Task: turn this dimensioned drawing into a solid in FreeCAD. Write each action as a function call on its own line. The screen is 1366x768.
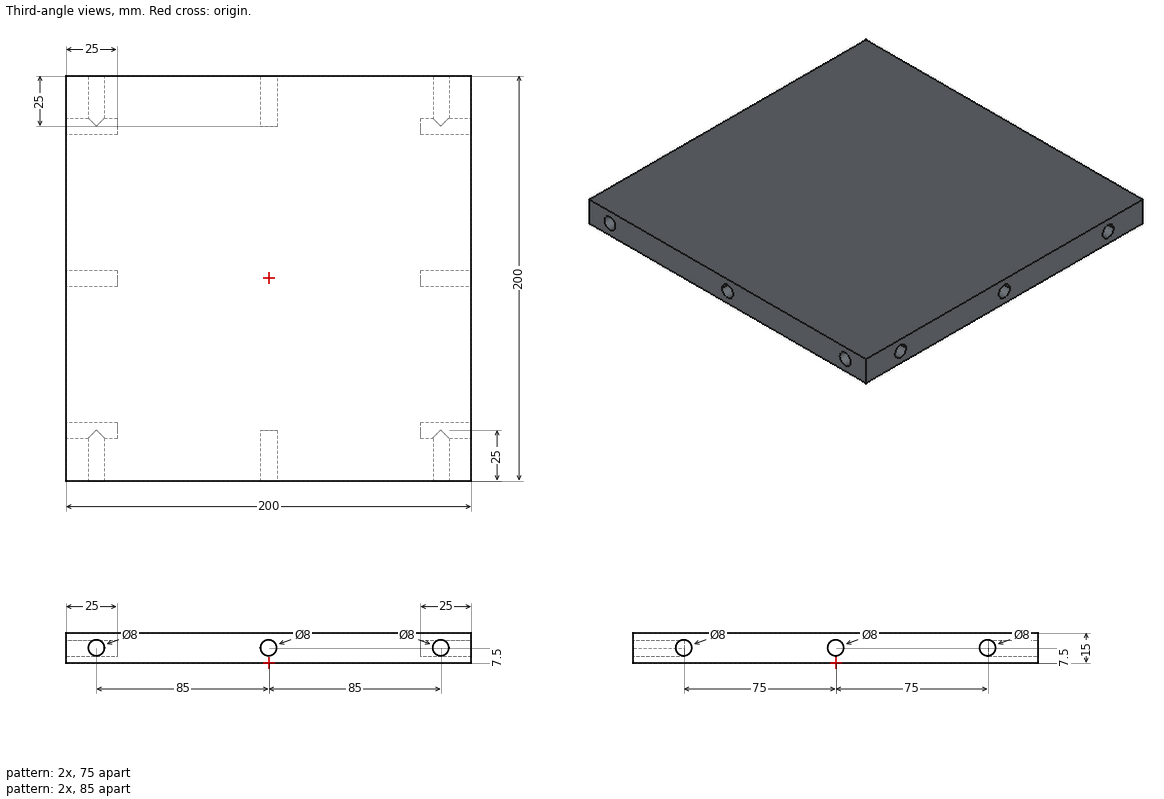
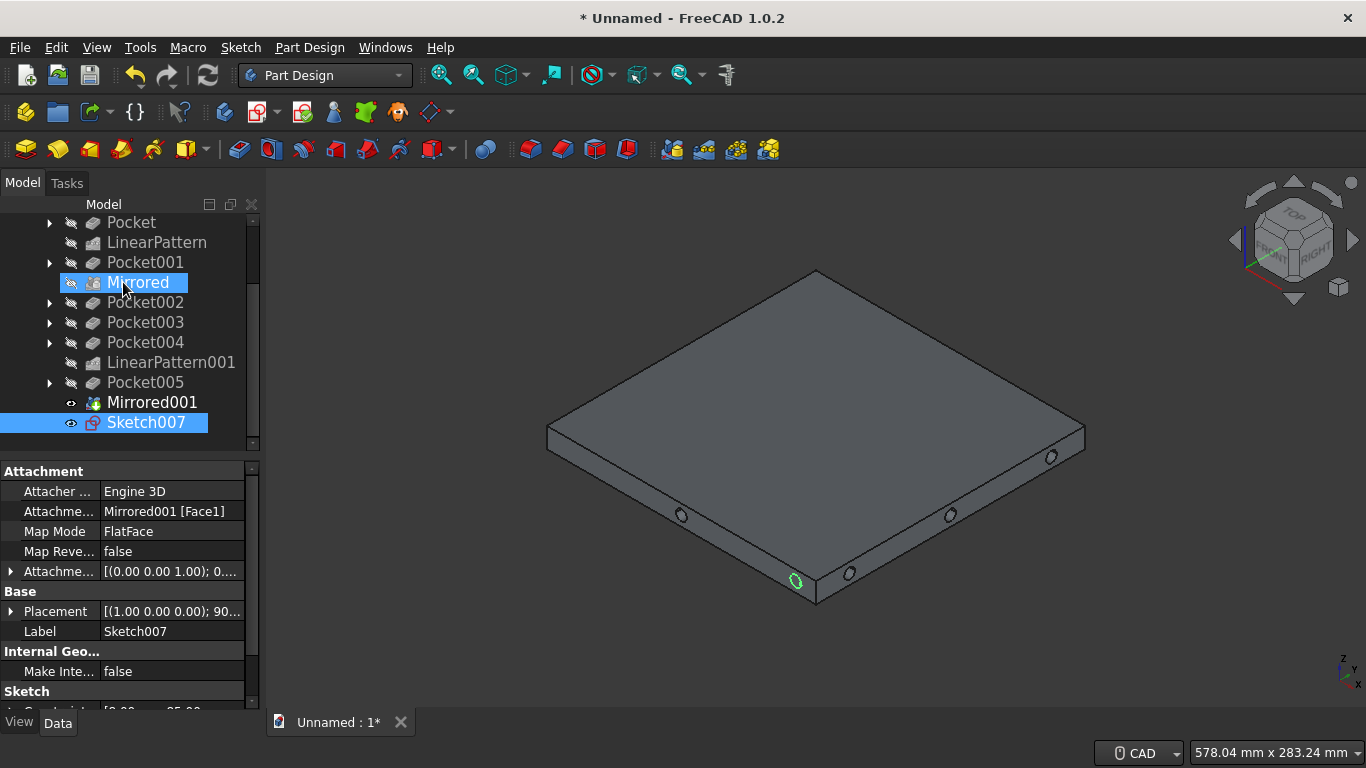
click(240, 150)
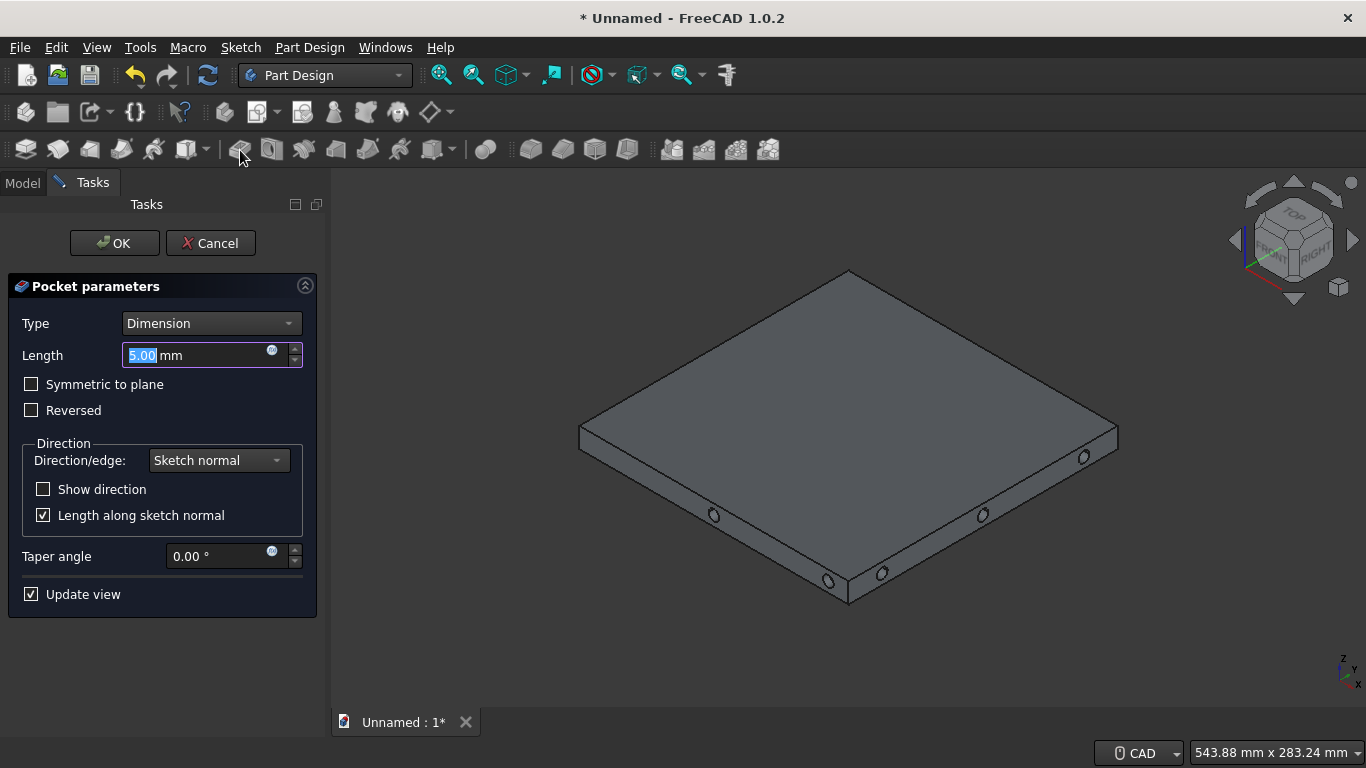
text(25)
key(Tab)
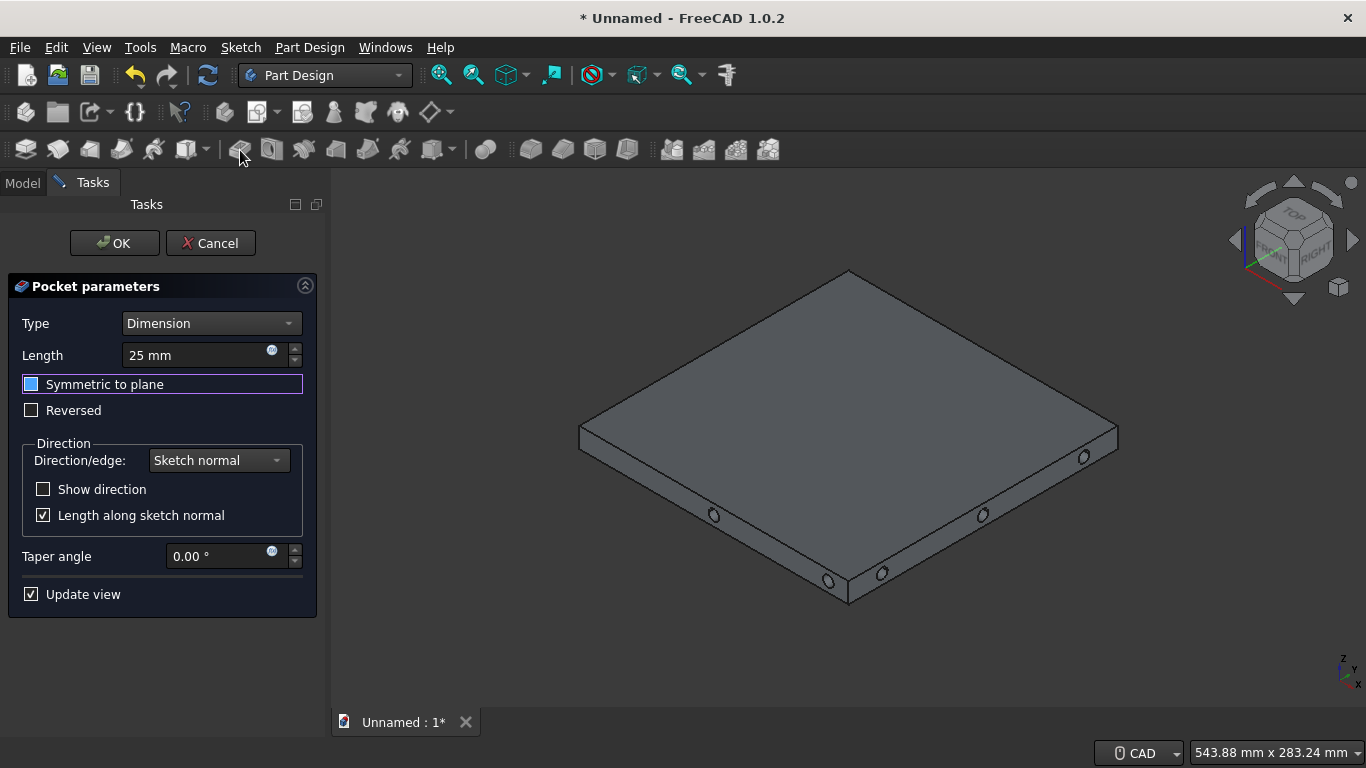
click(115, 243)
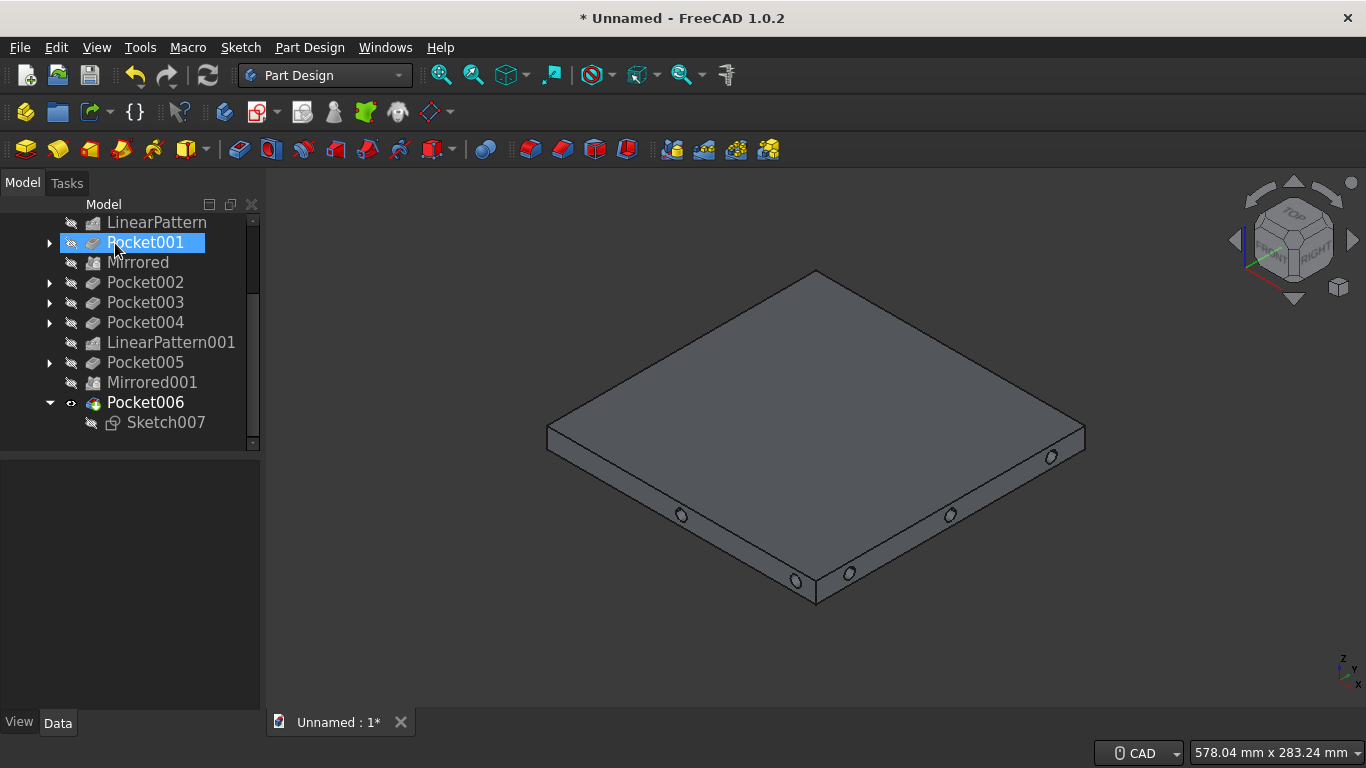
click(758, 559)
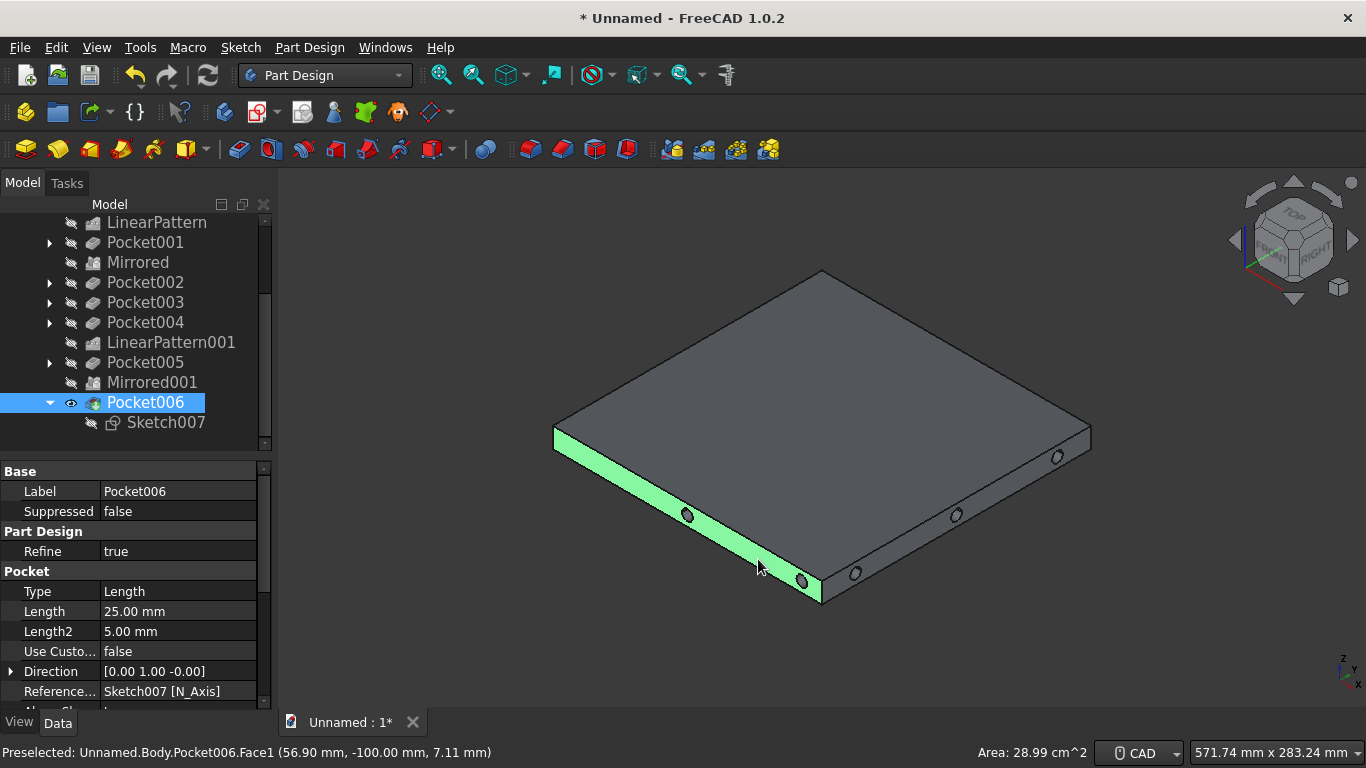
click(258, 112)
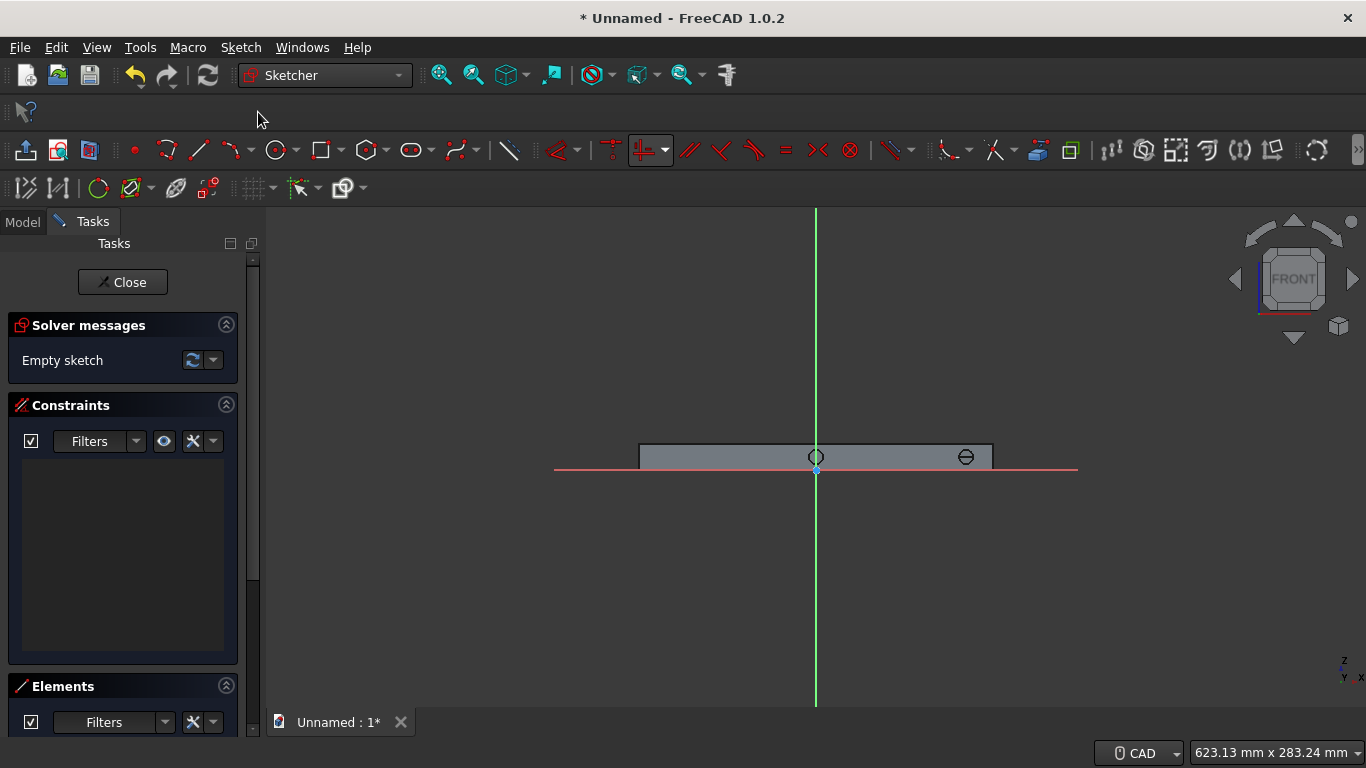
scroll(662, 457, up, 15)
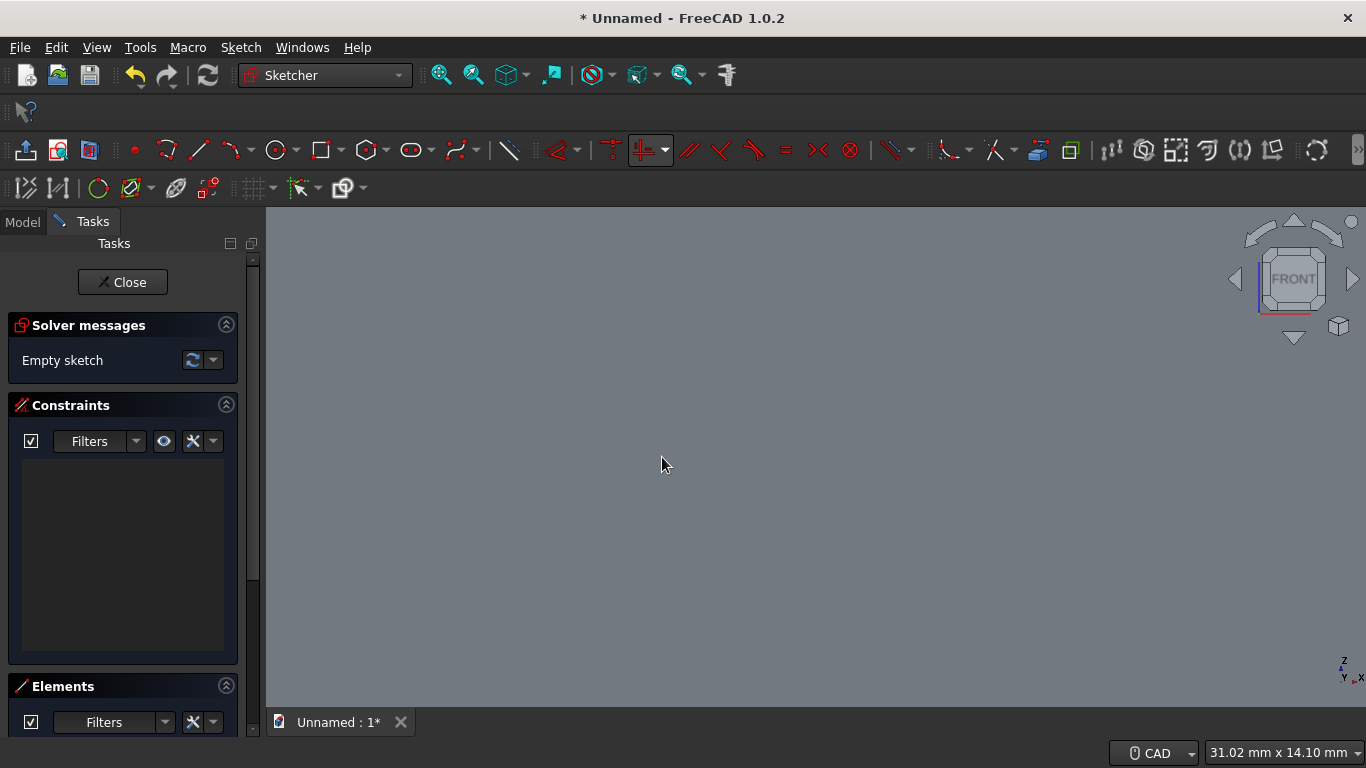
key(g)
key(c)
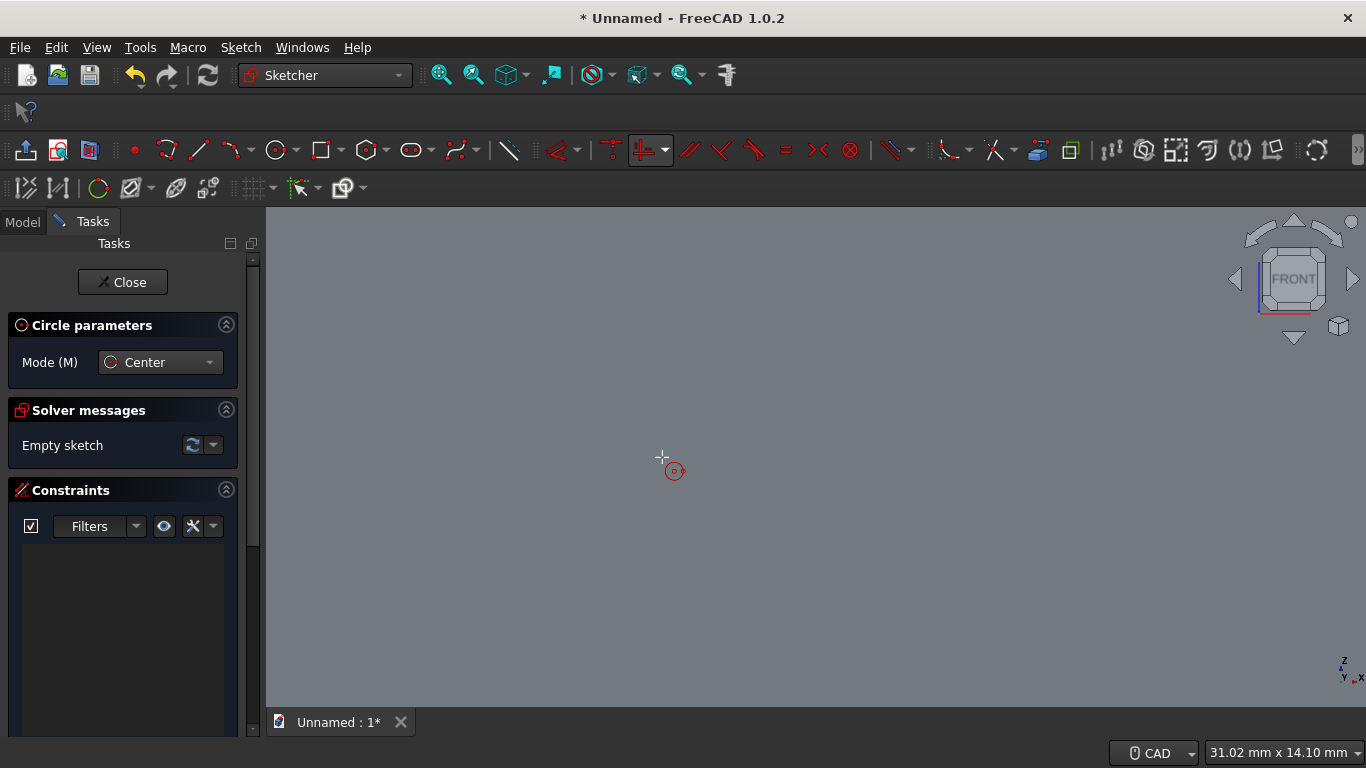
click(734, 447)
move(835, 347)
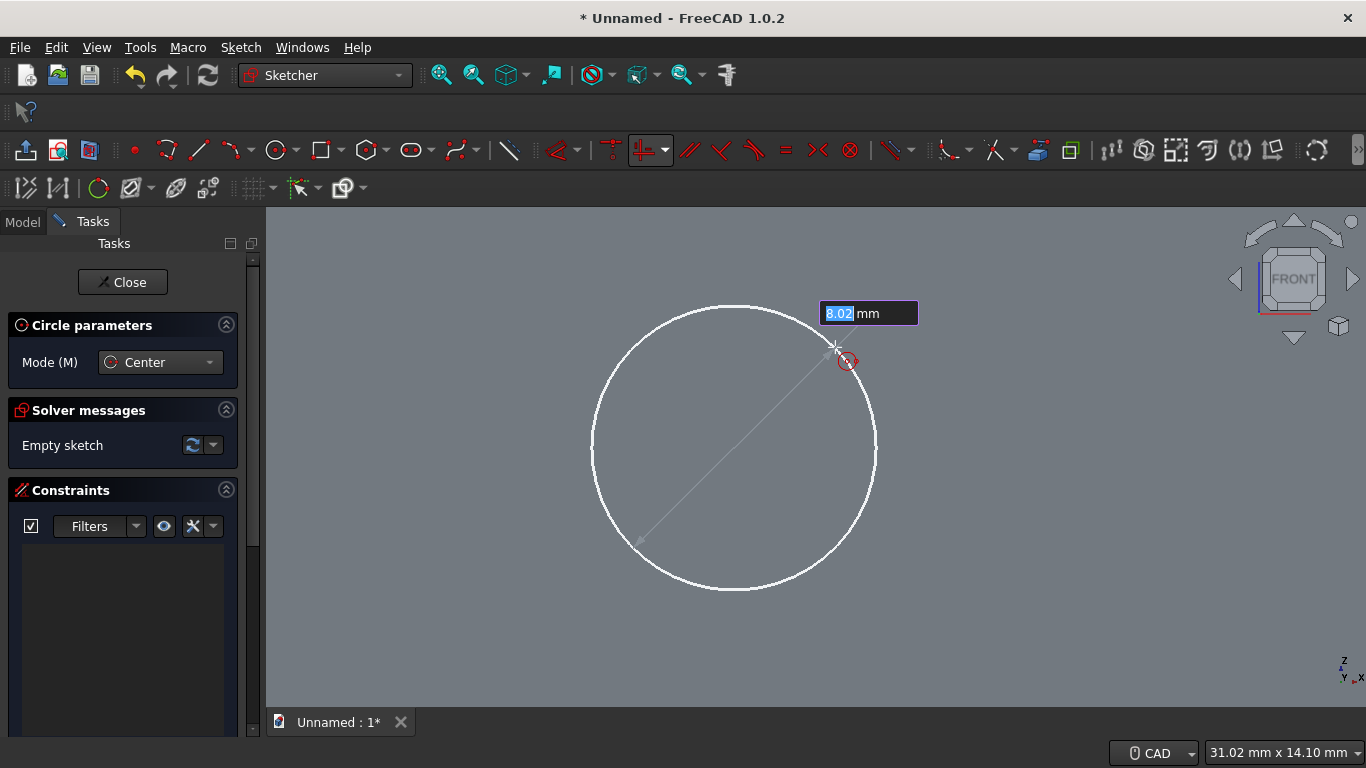
text(8)
key(Return)
key(Escape)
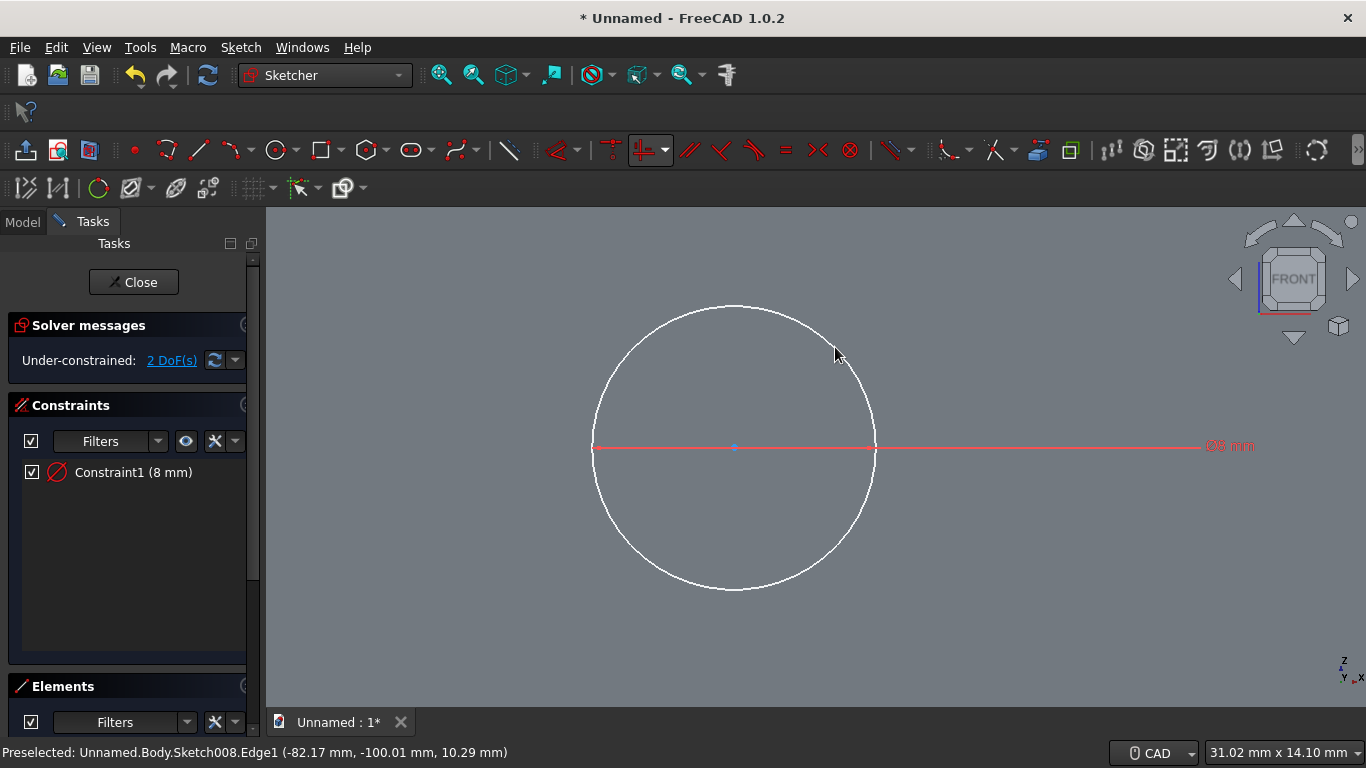
key(d)